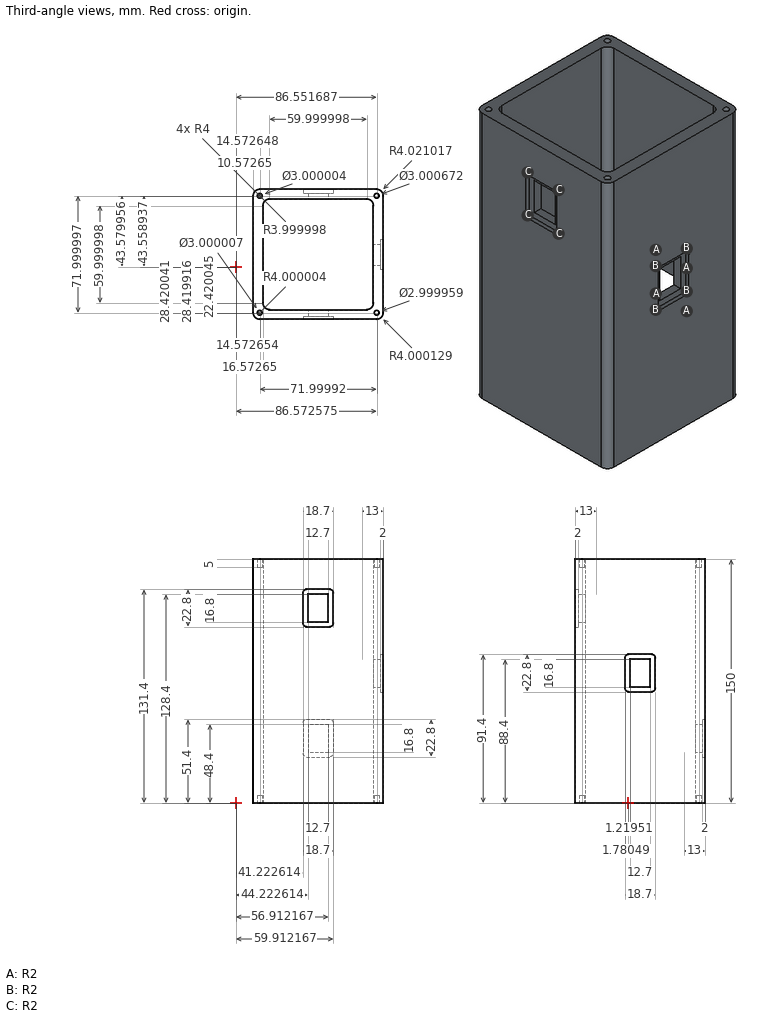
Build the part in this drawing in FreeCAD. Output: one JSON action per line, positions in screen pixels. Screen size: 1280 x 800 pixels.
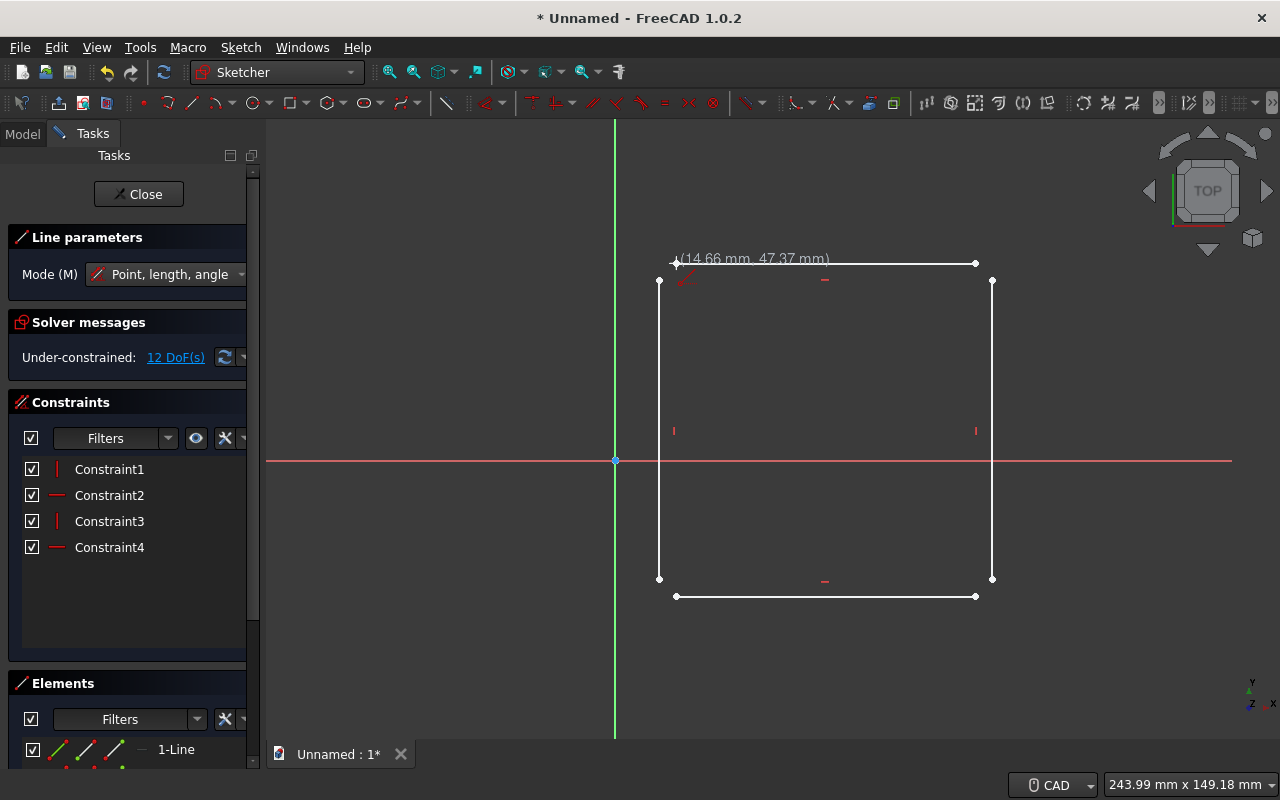
{"action": "key", "text": "g 3 a"}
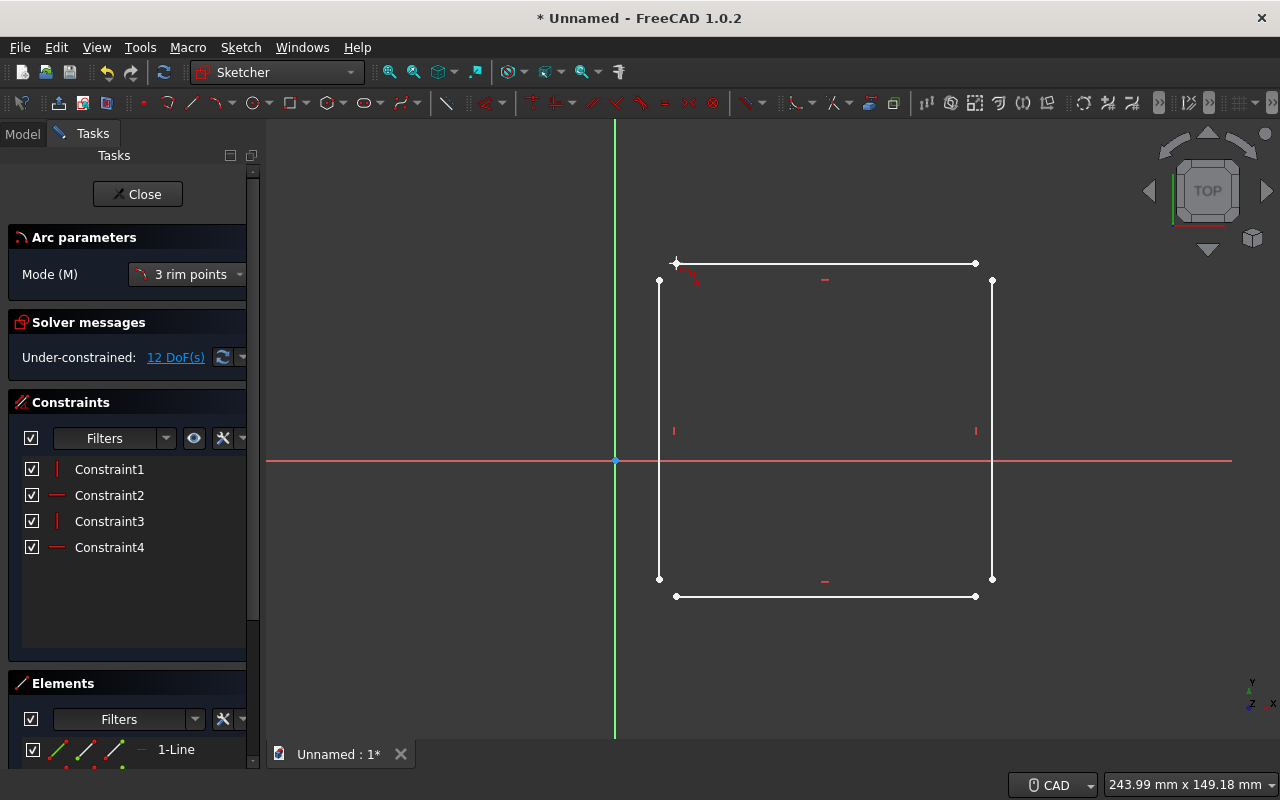
{"action": "left_click", "coordinate": [659, 580]}
{"action": "left_click", "coordinate": [676, 597]}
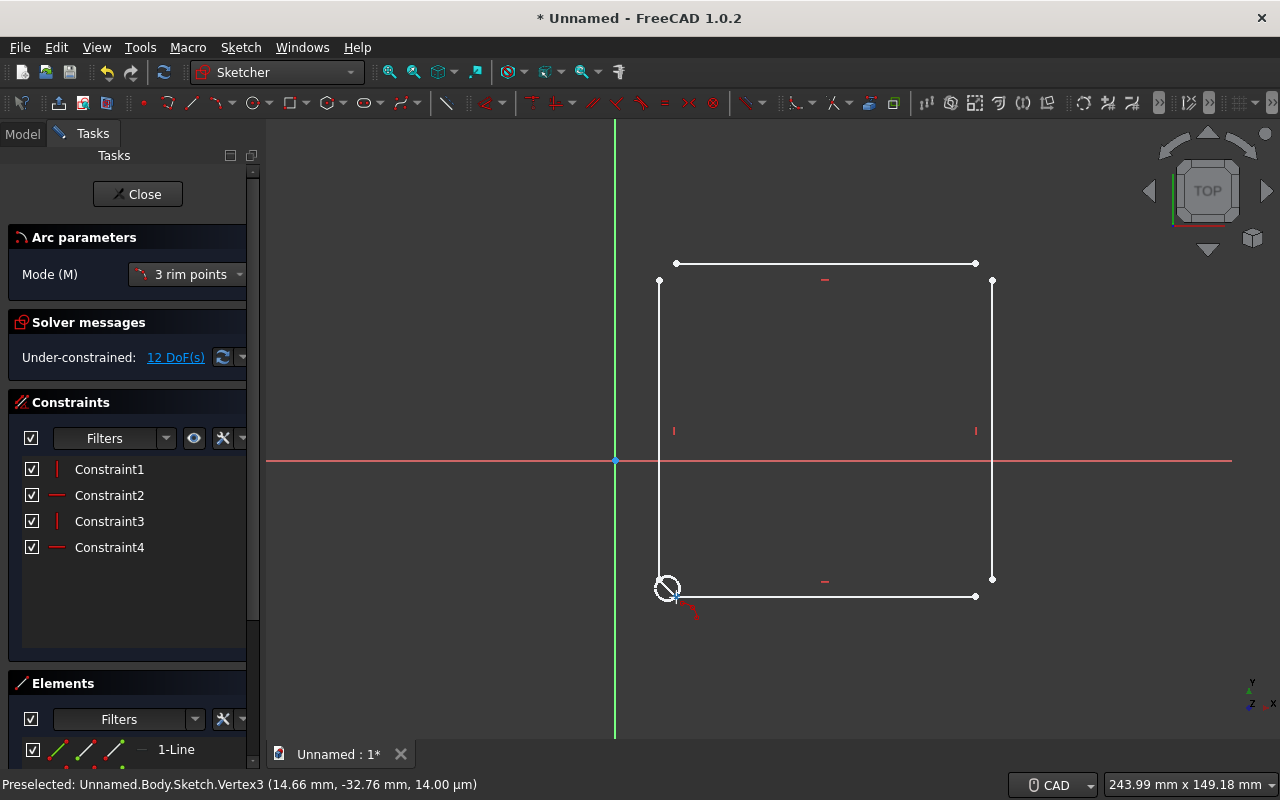
{"action": "scroll", "coordinate": [664, 591], "scroll_direction": "up", "scroll_amount": 6}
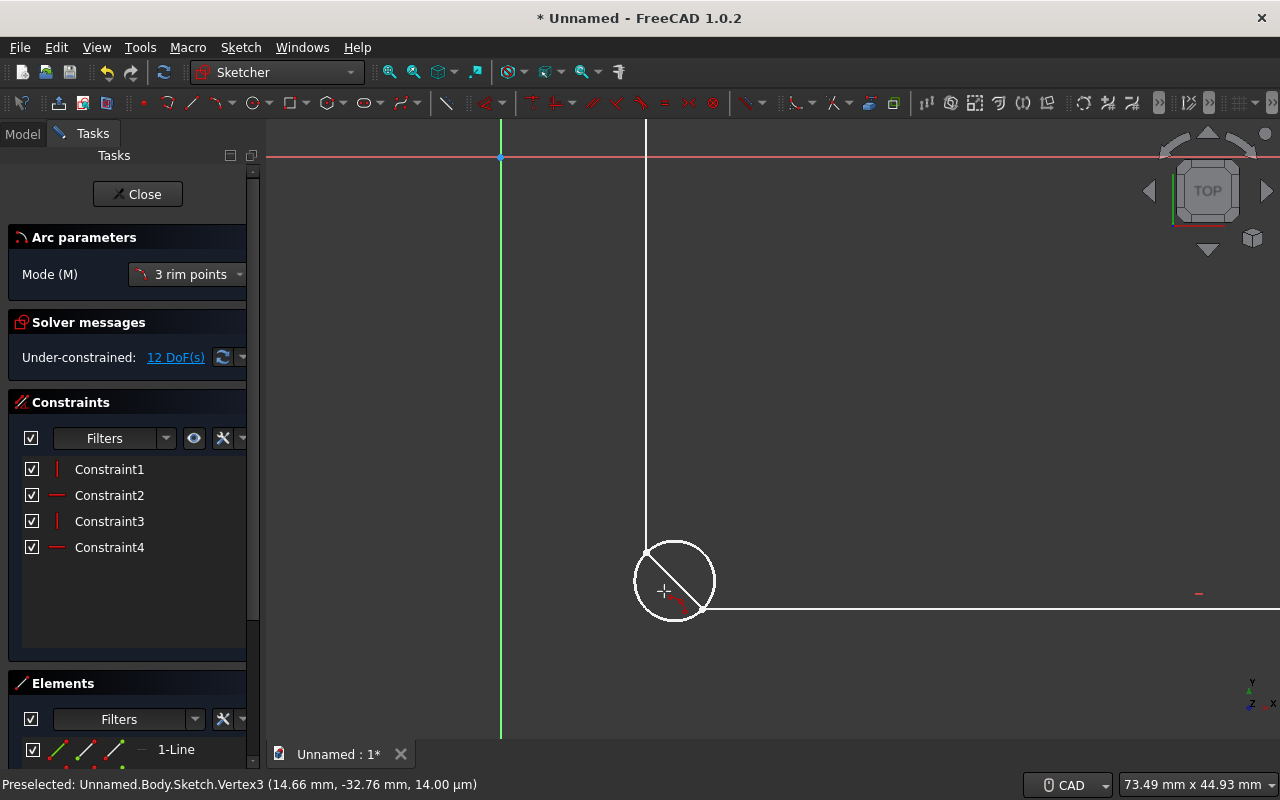
{"action": "left_click", "coordinate": [663, 588]}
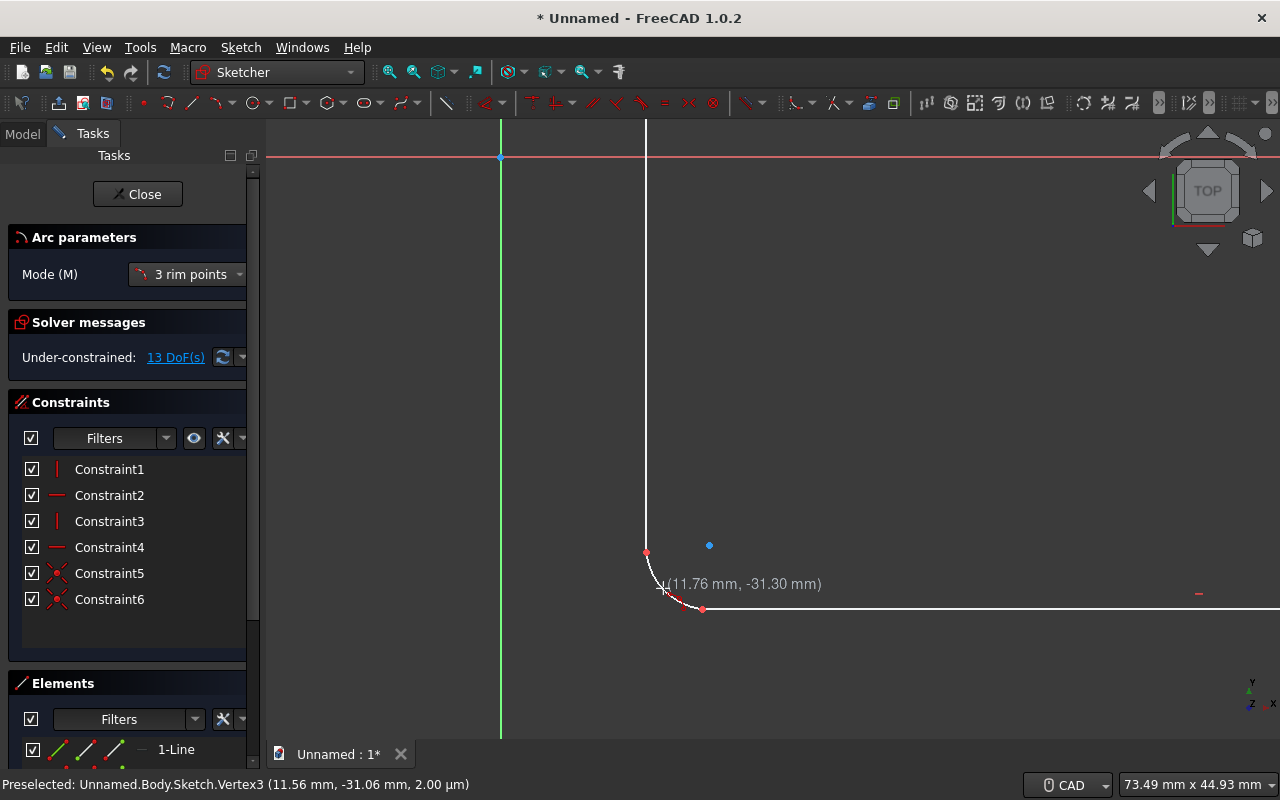
{"action": "scroll", "coordinate": [459, 648], "scroll_direction": "down", "scroll_amount": 5}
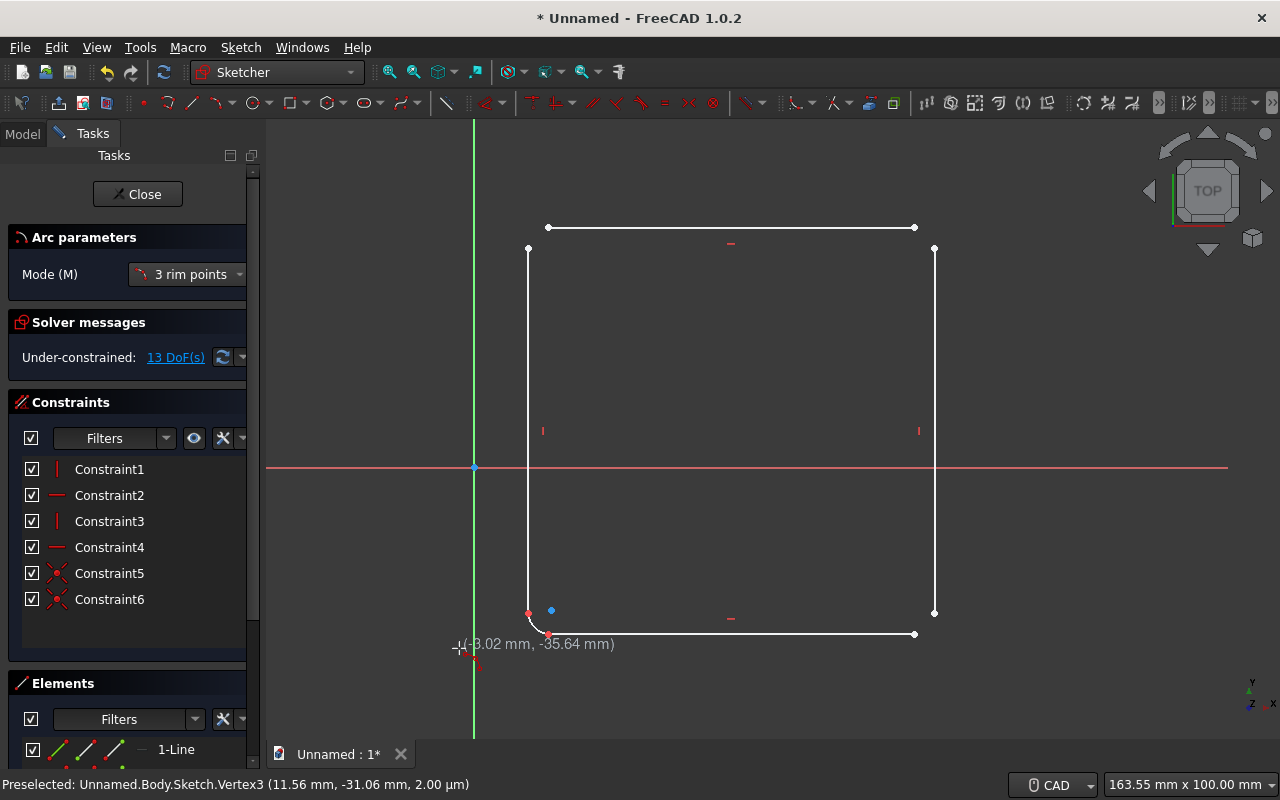
{"action": "left_click", "coordinate": [914, 634]}
{"action": "left_click", "coordinate": [935, 613]}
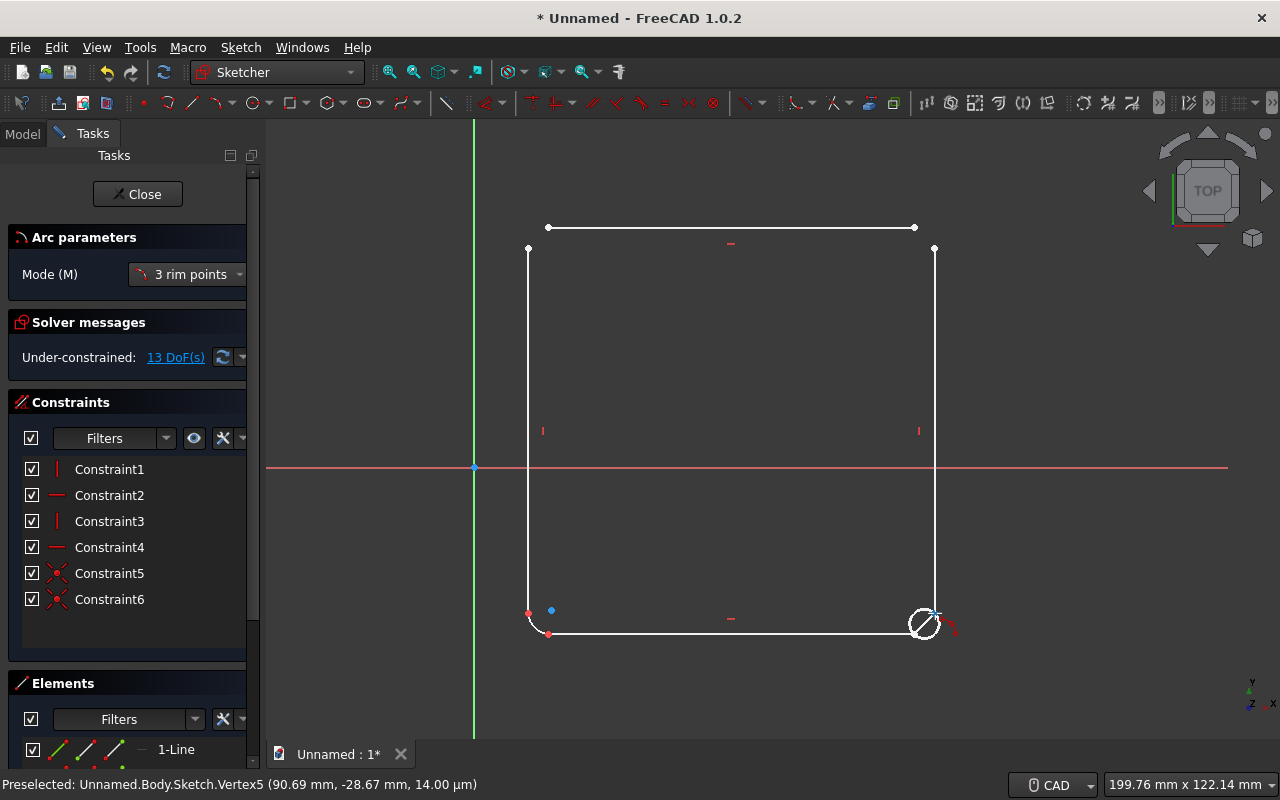
{"action": "scroll", "coordinate": [928, 627], "scroll_direction": "up", "scroll_amount": 5}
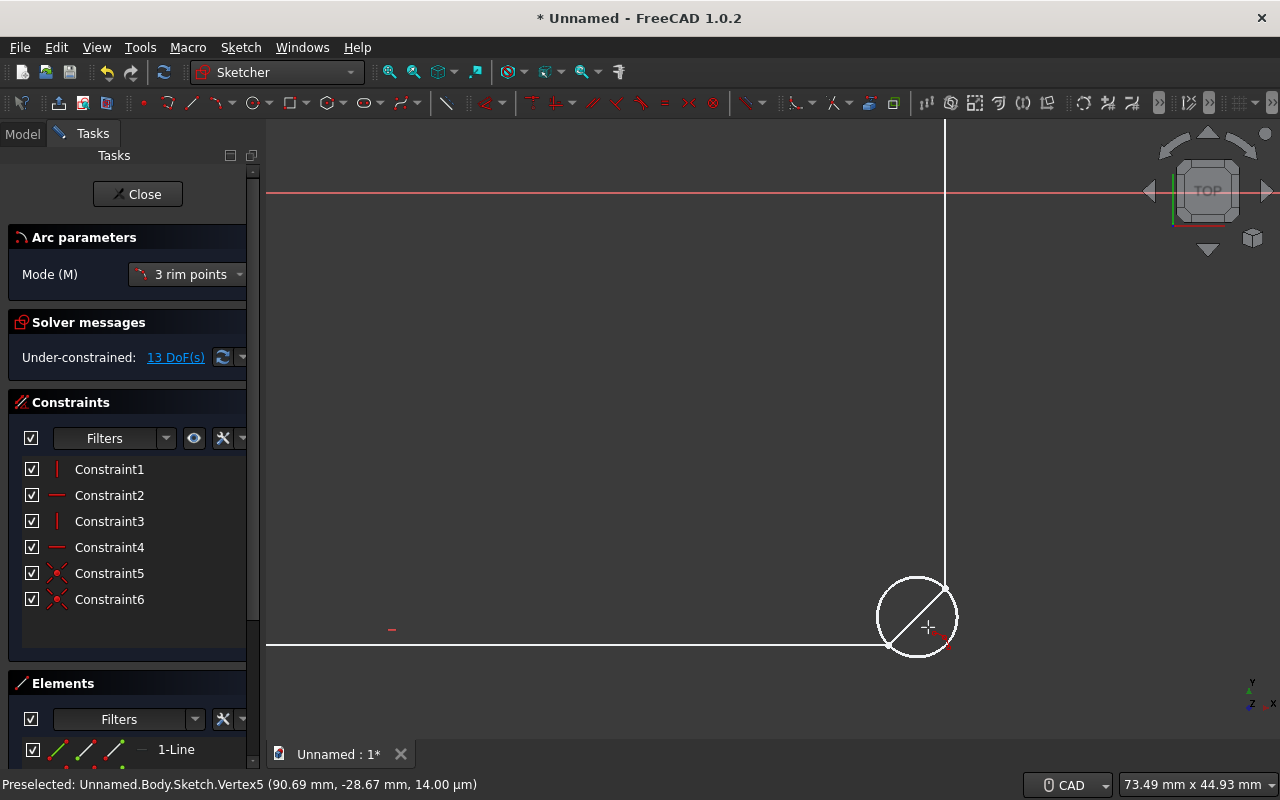
{"action": "left_click", "coordinate": [928, 624]}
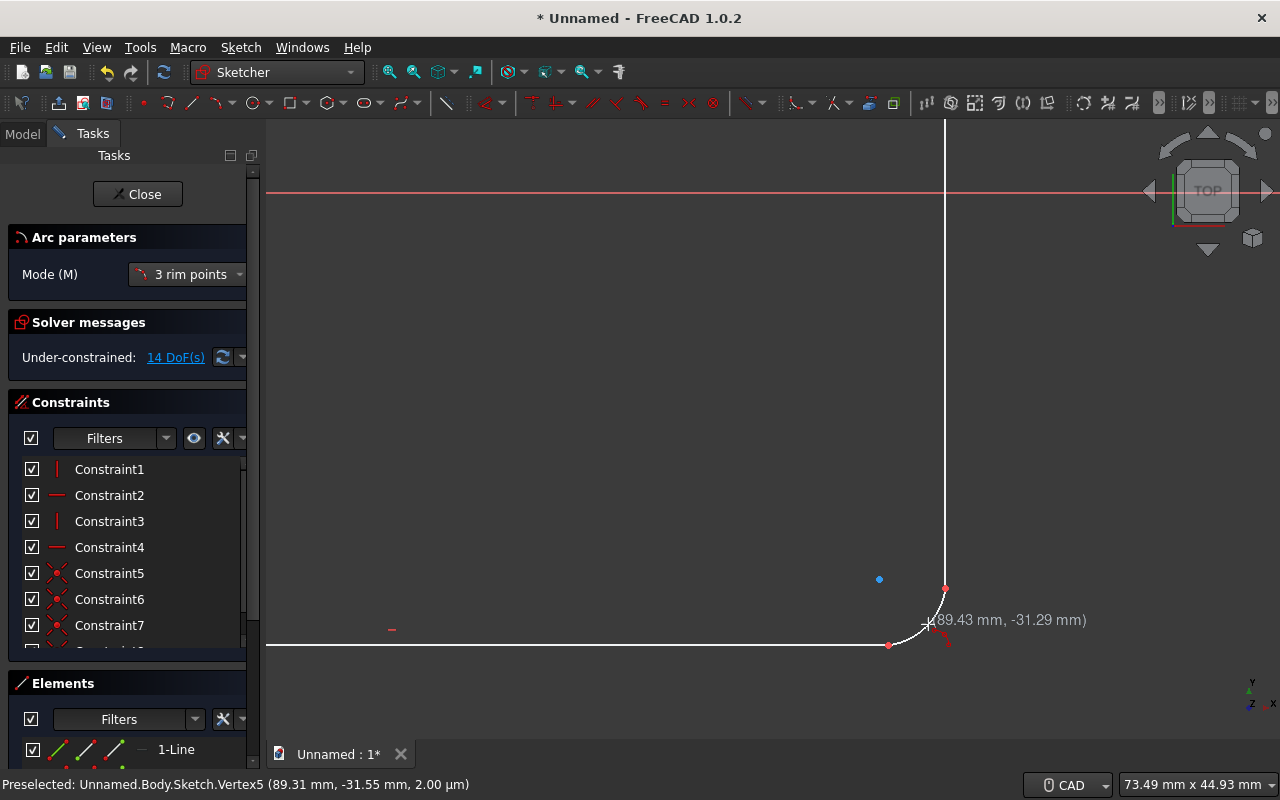
{"action": "scroll", "coordinate": [929, 627], "scroll_direction": "down", "scroll_amount": 5}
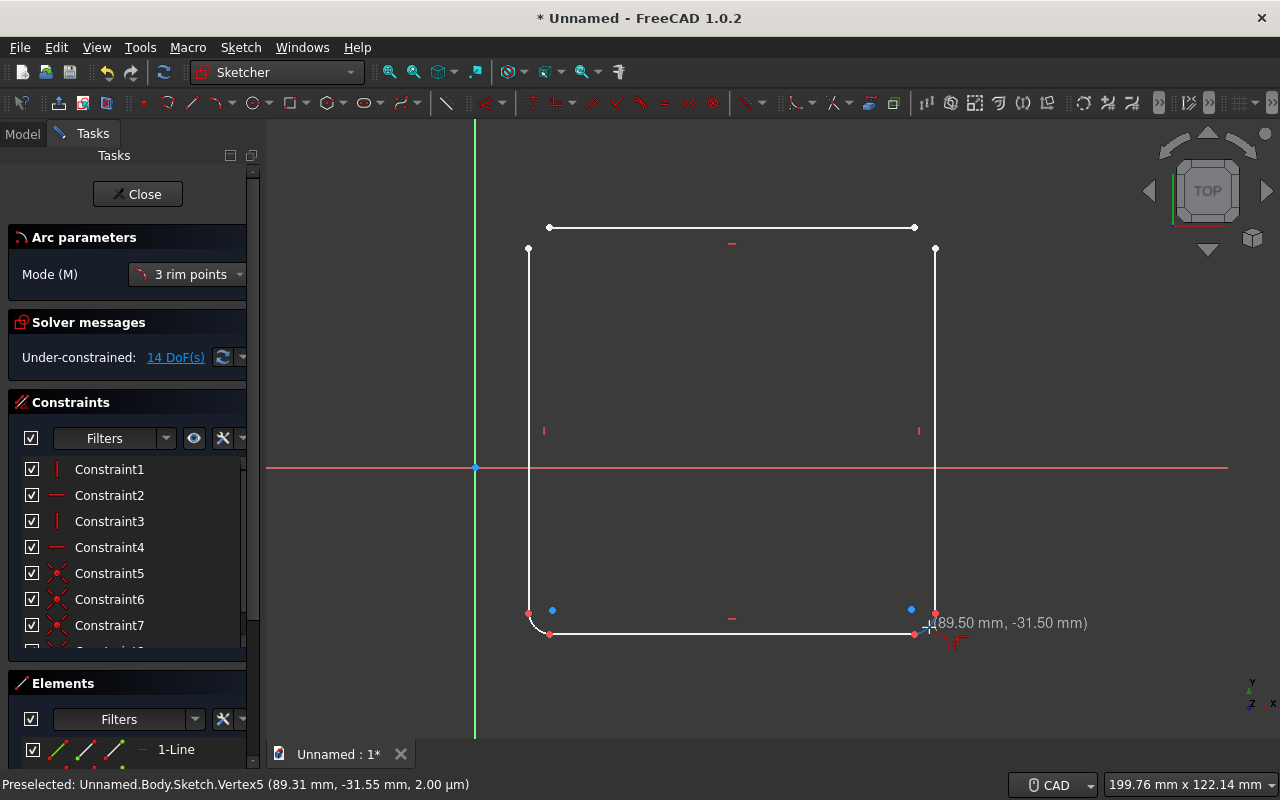
{"action": "left_click", "coordinate": [935, 248]}
{"action": "left_click", "coordinate": [915, 228]}